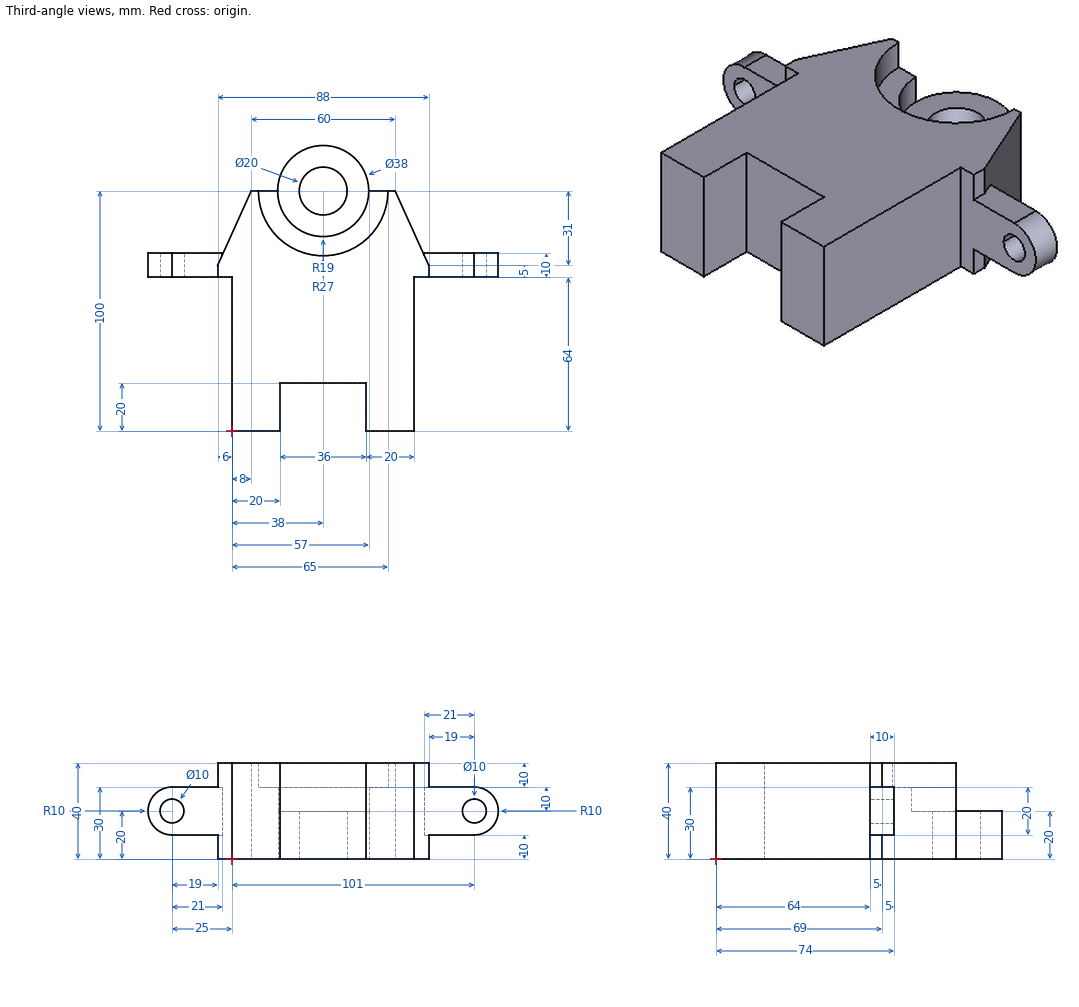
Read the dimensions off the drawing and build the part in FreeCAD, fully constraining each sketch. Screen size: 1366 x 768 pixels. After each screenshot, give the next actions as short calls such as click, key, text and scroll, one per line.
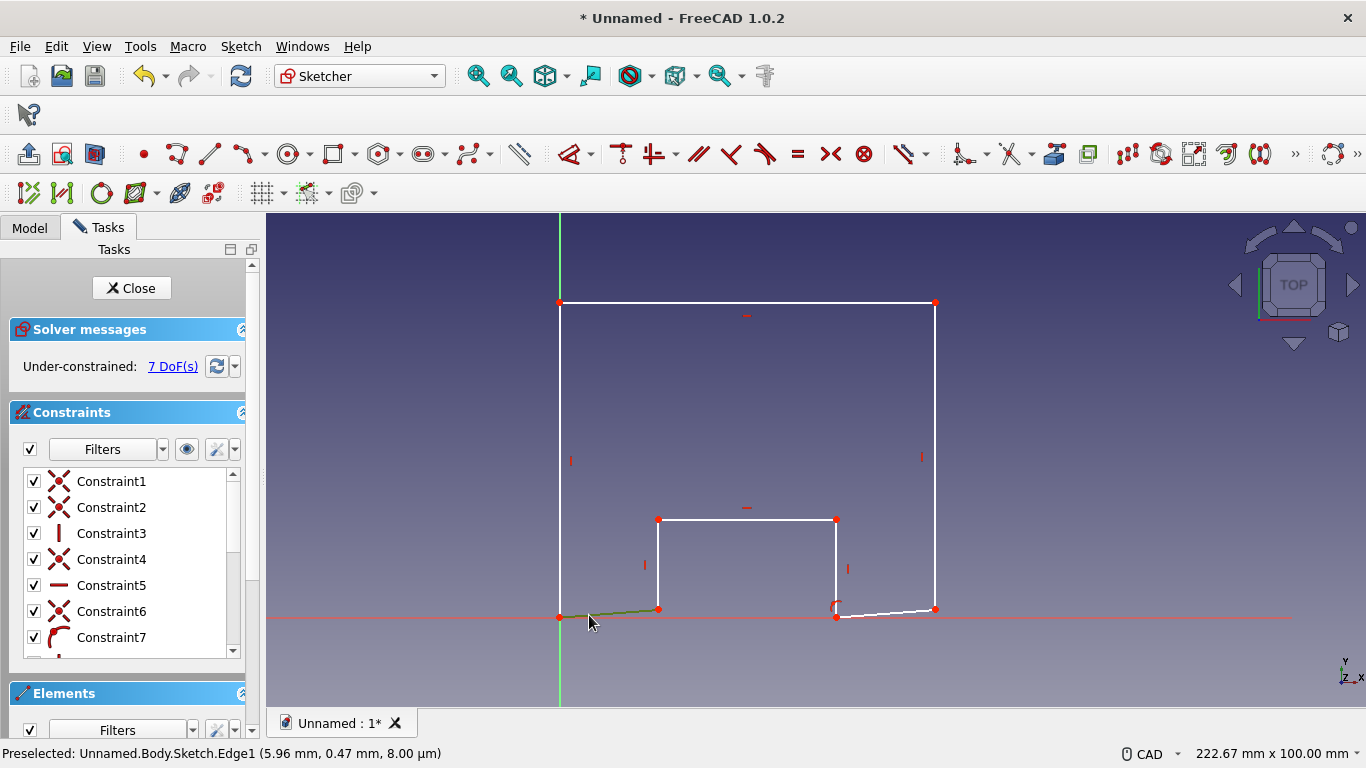
key(h)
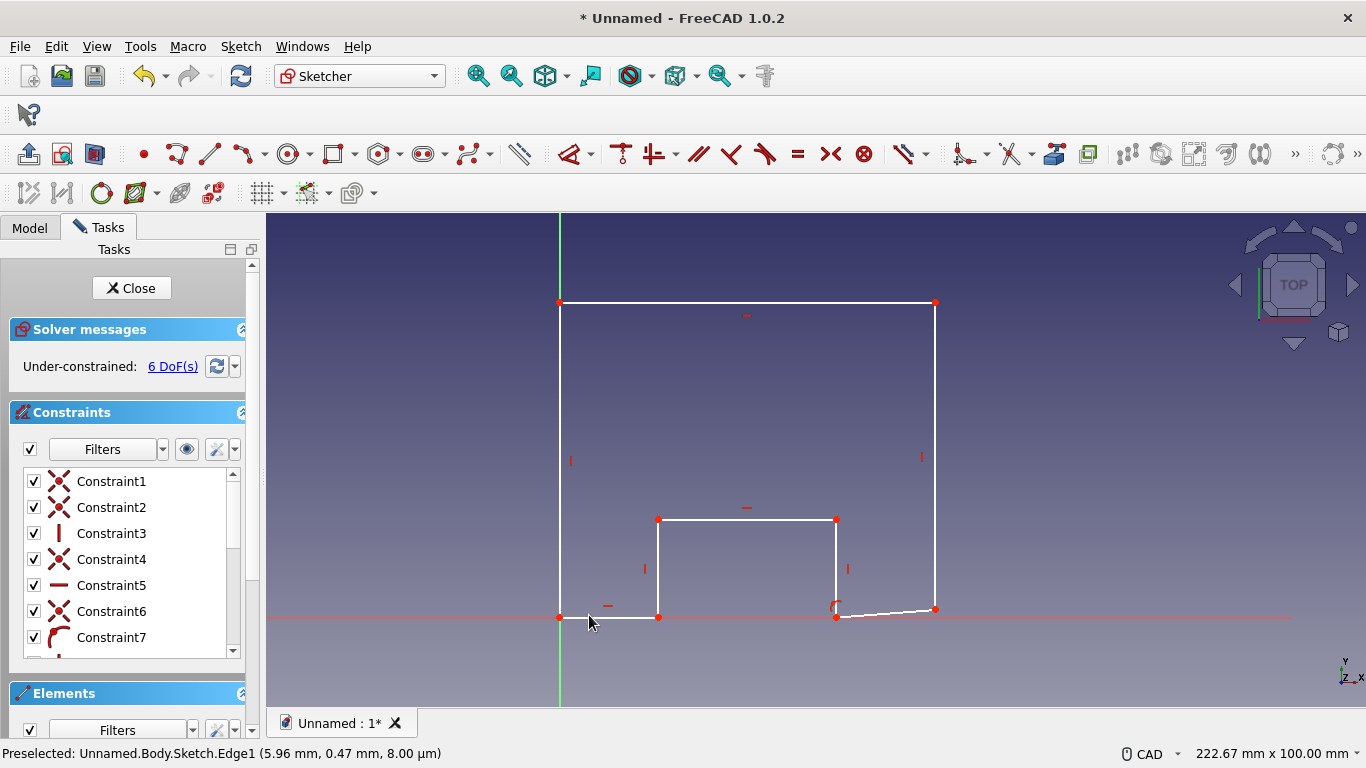
click(866, 615)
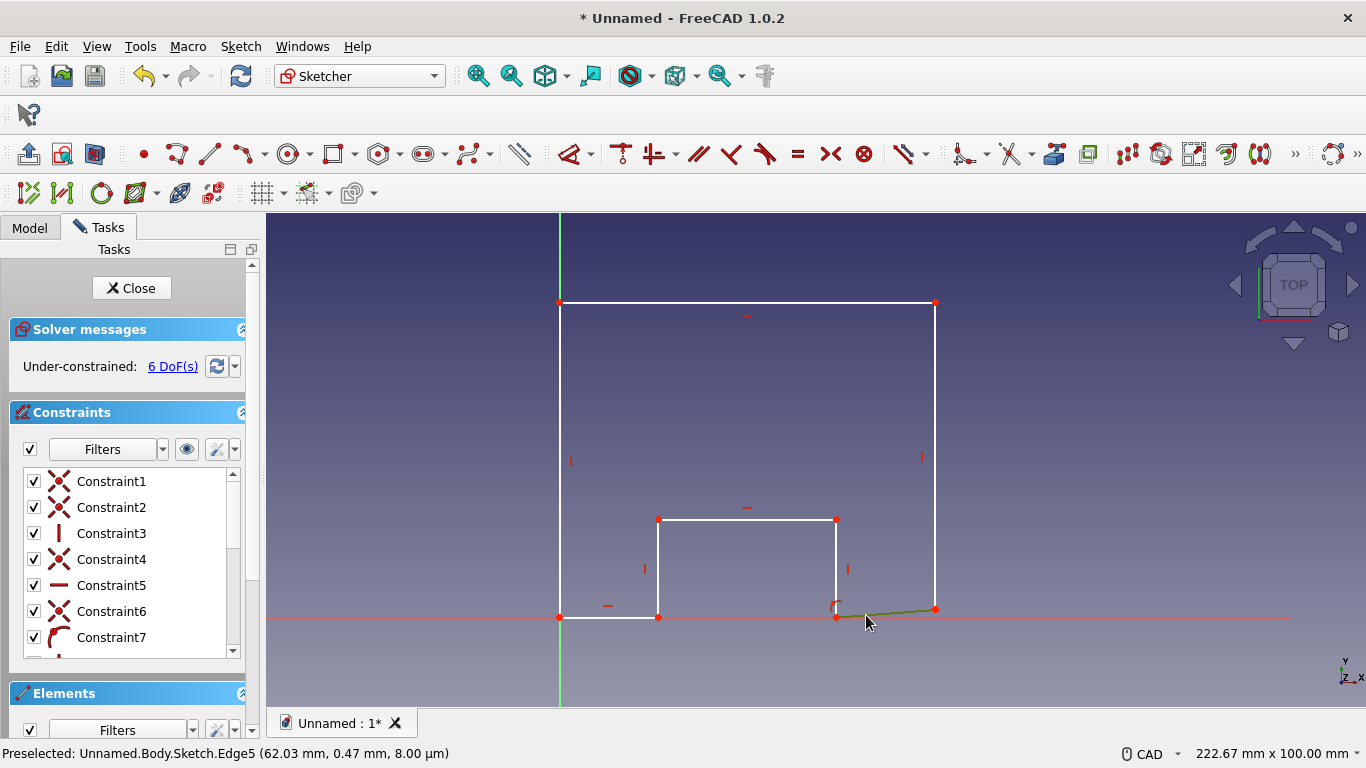
click(676, 154)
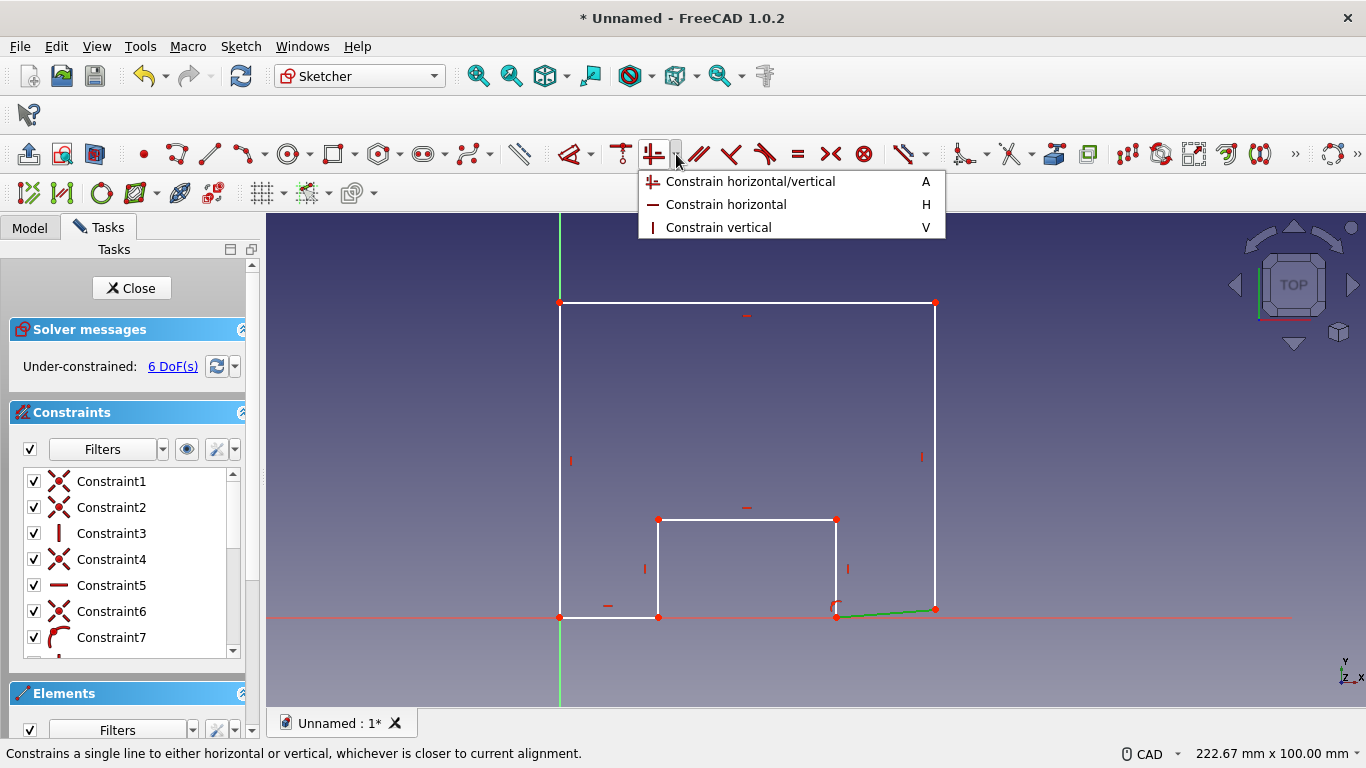
click(792, 204)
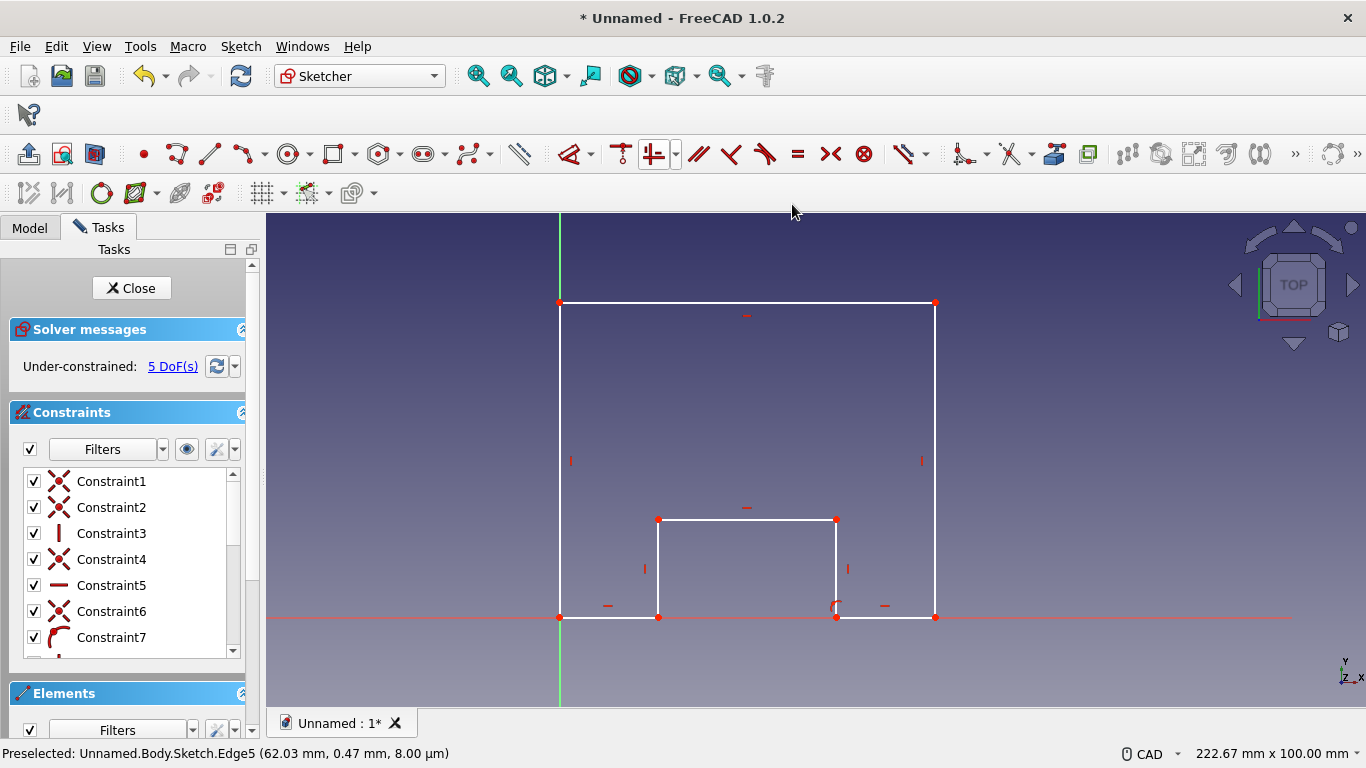
click(568, 154)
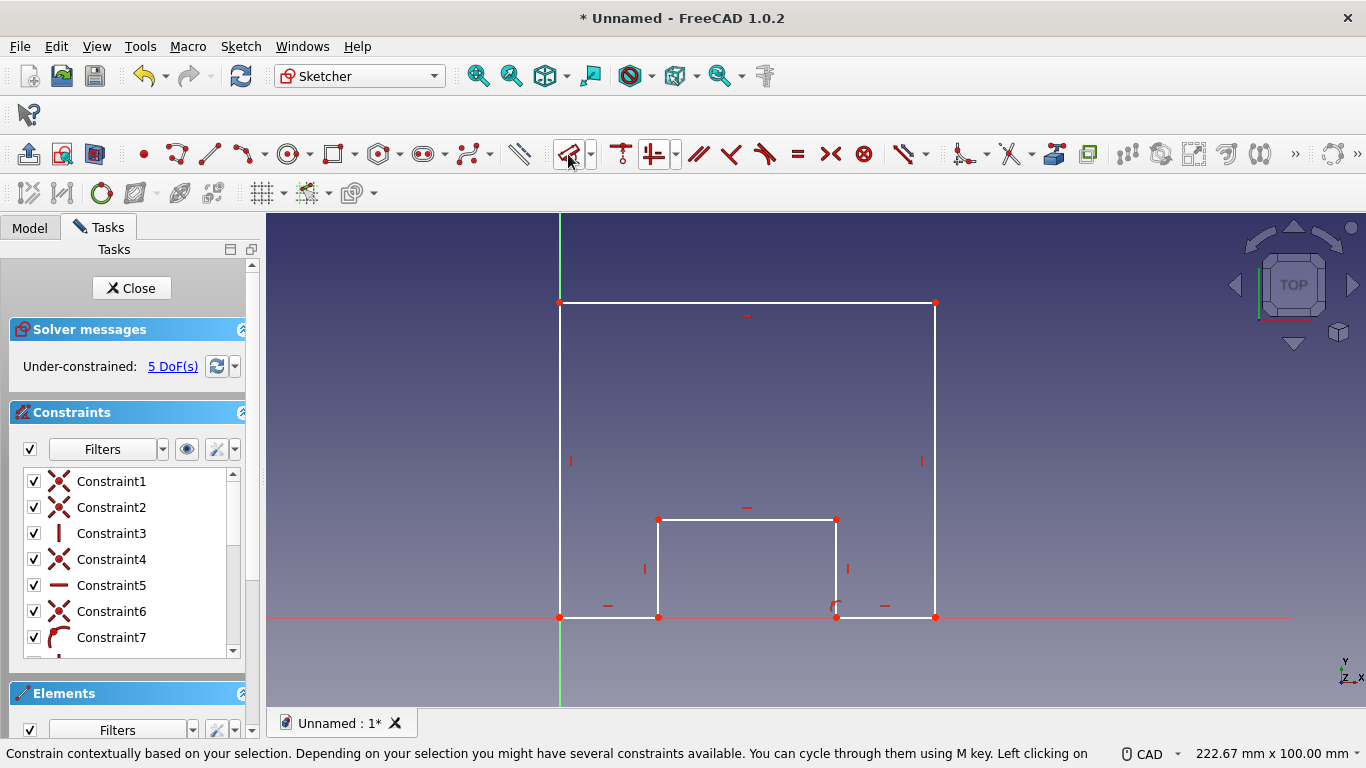
click(589, 618)
click(609, 652)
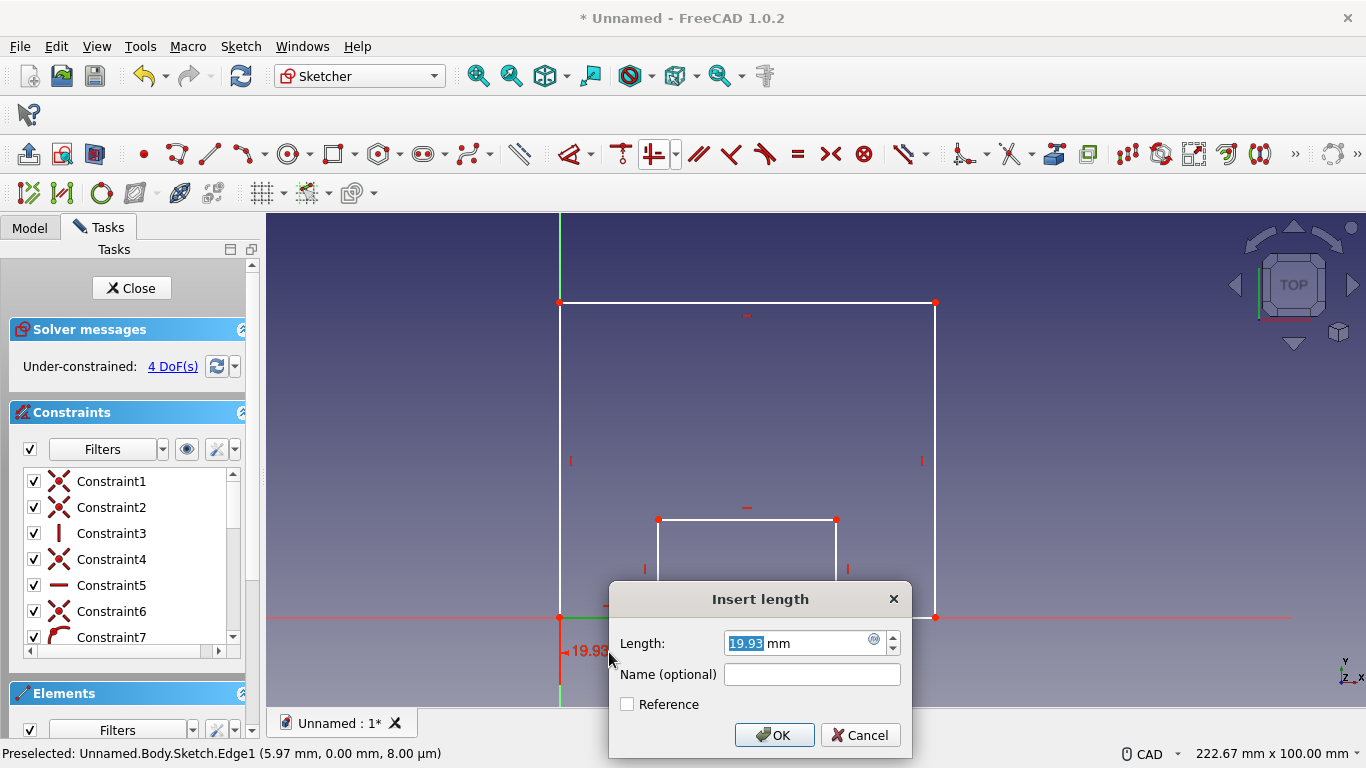
text(20)
key(Return)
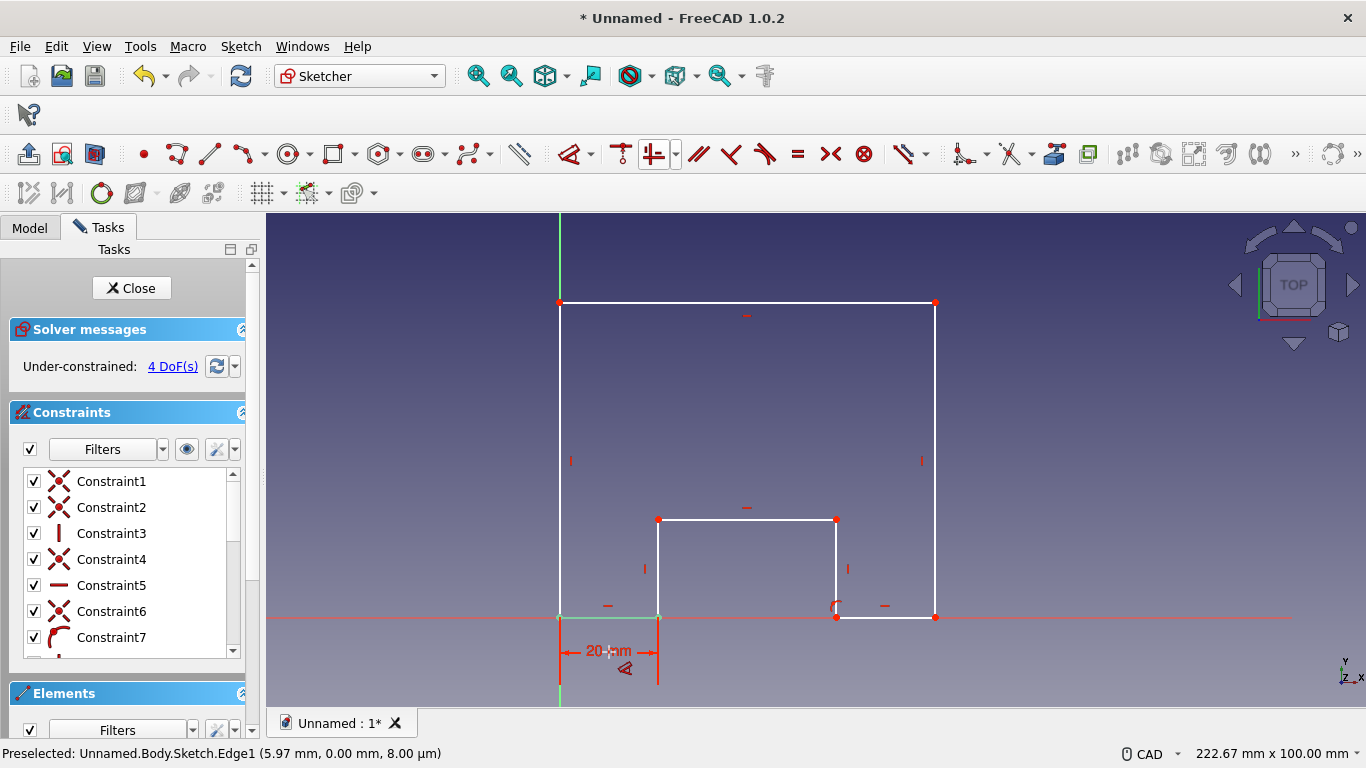
click(658, 588)
click(624, 569)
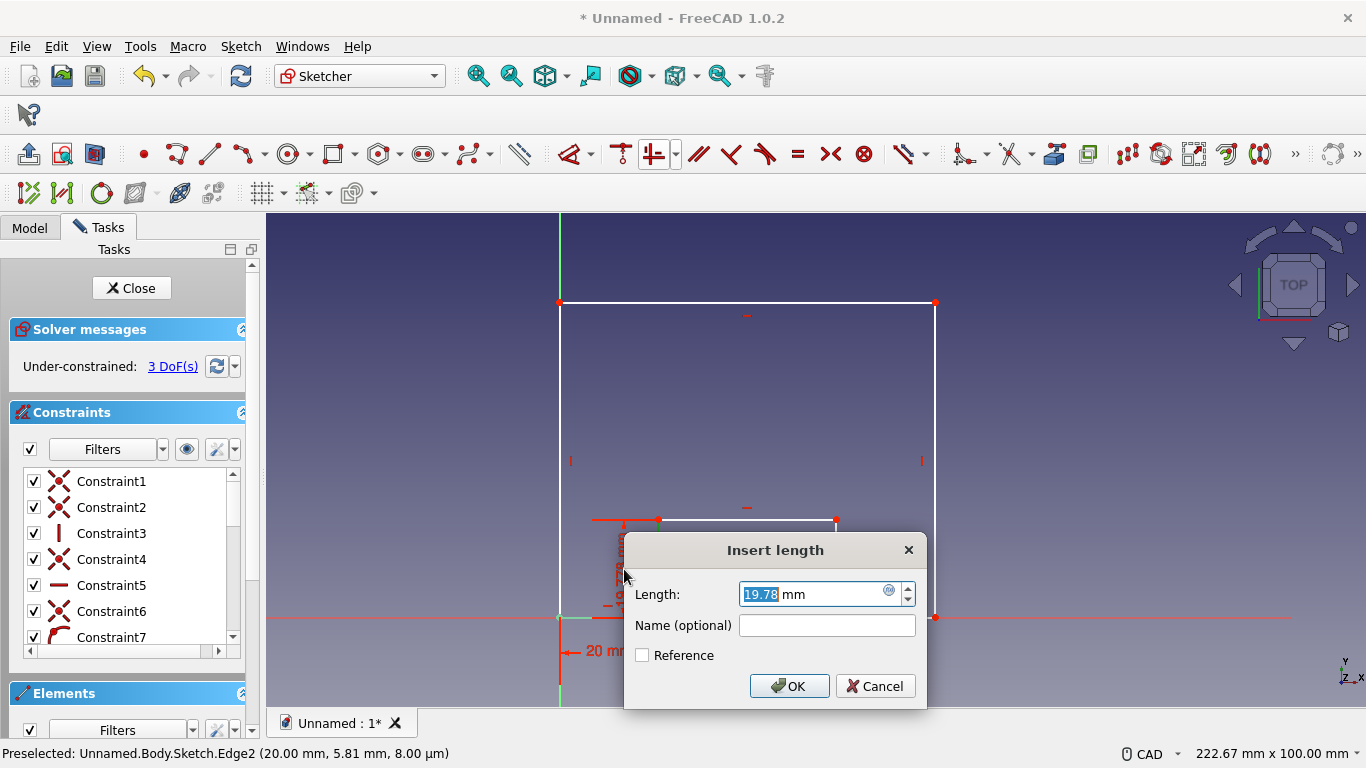
text(20)
key(Return)